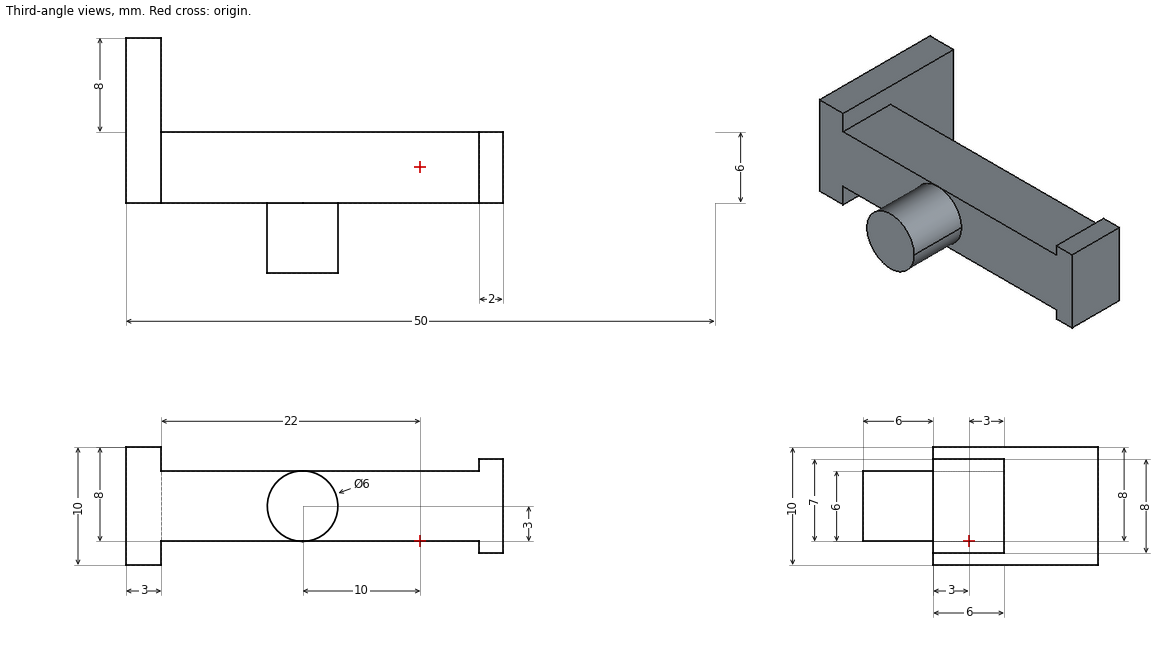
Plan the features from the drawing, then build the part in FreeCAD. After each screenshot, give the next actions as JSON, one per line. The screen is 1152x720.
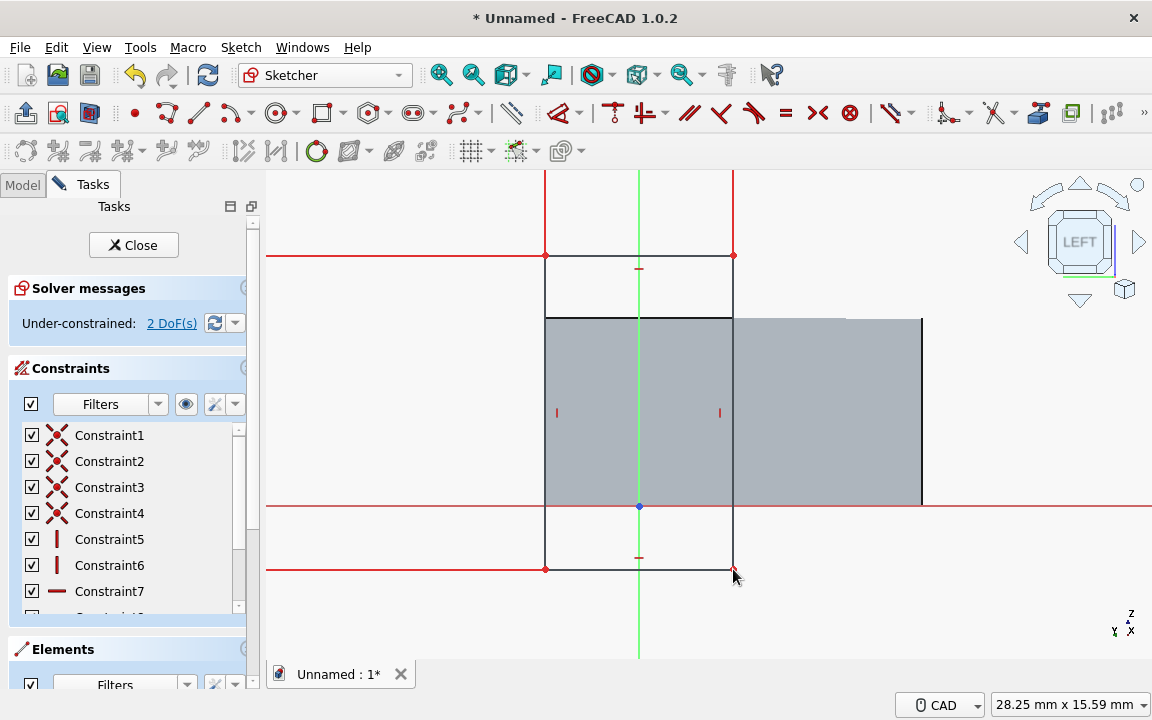
{"action": "left_click", "coordinate": [558, 114]}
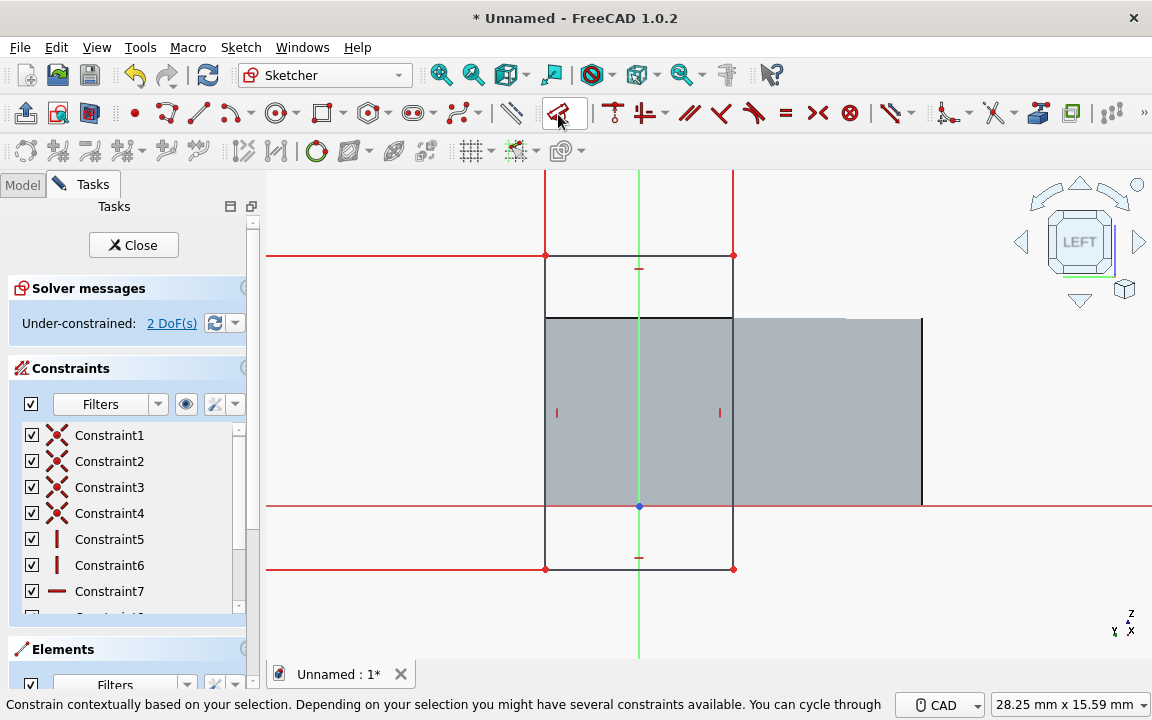
{"action": "left_click", "coordinate": [545, 256]}
{"action": "left_click", "coordinate": [592, 222]}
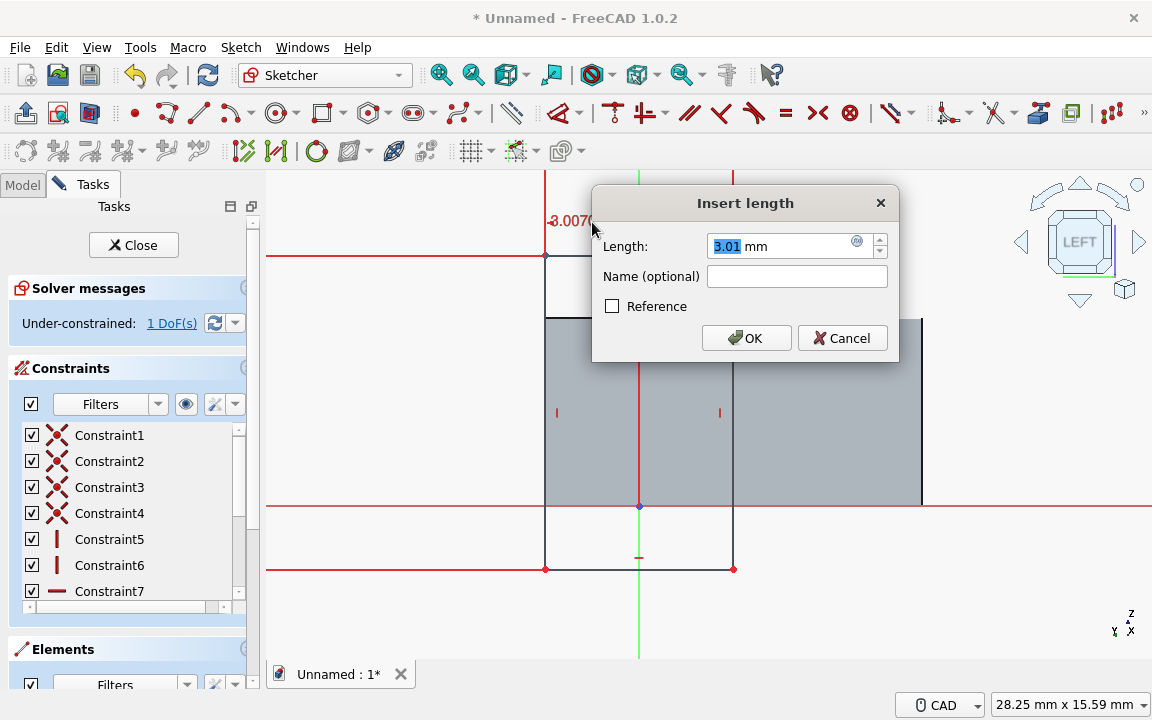
{"action": "type", "text": "3"}
{"action": "key", "text": "Return"}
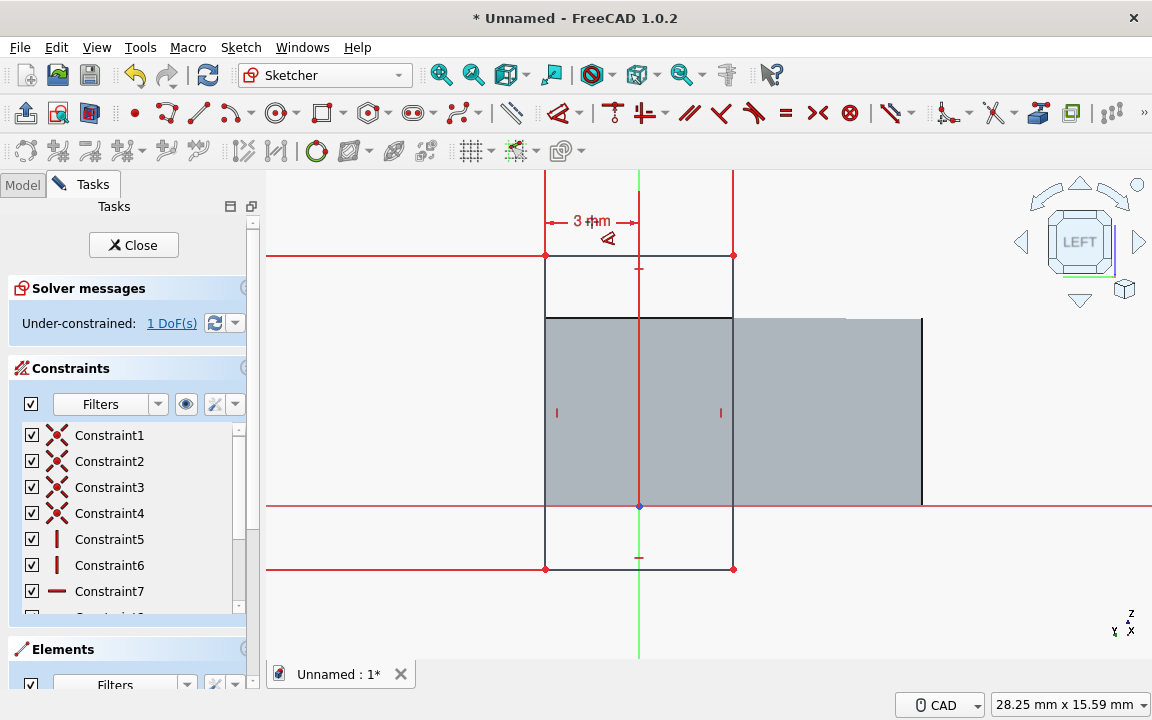
{"action": "left_click", "coordinate": [545, 256]}
{"action": "left_click", "coordinate": [511, 381]}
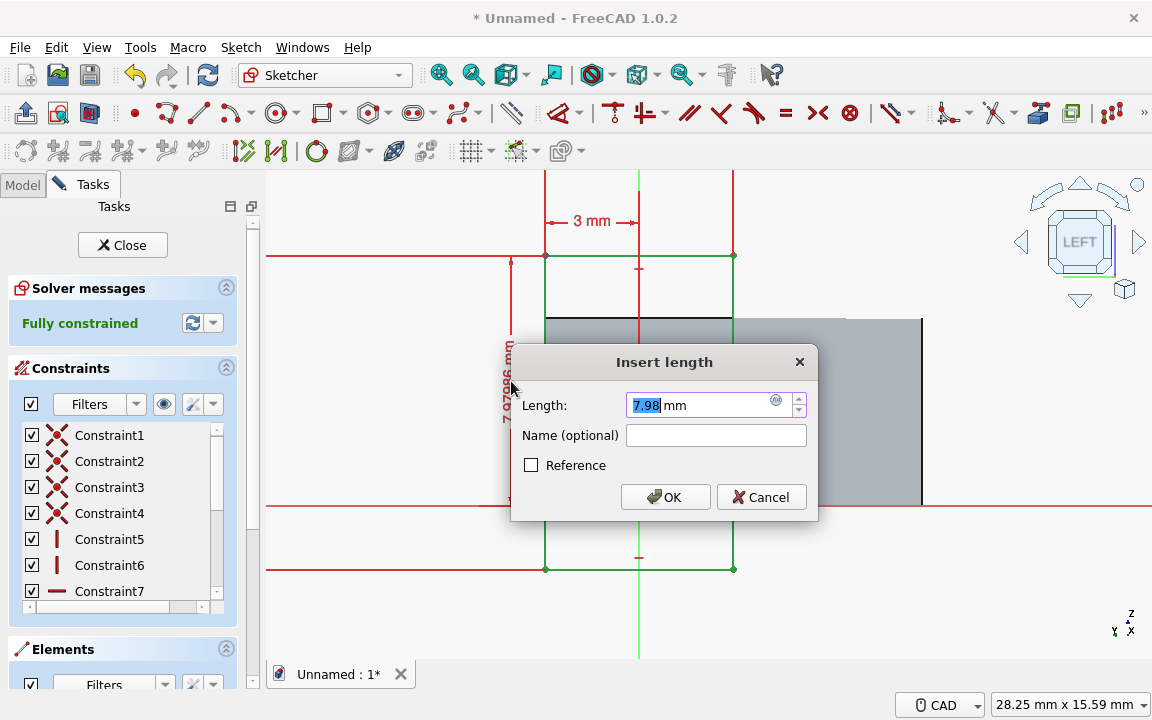
{"action": "type", "text": "8"}
{"action": "key", "text": "Return"}
{"action": "key", "text": "Escape"}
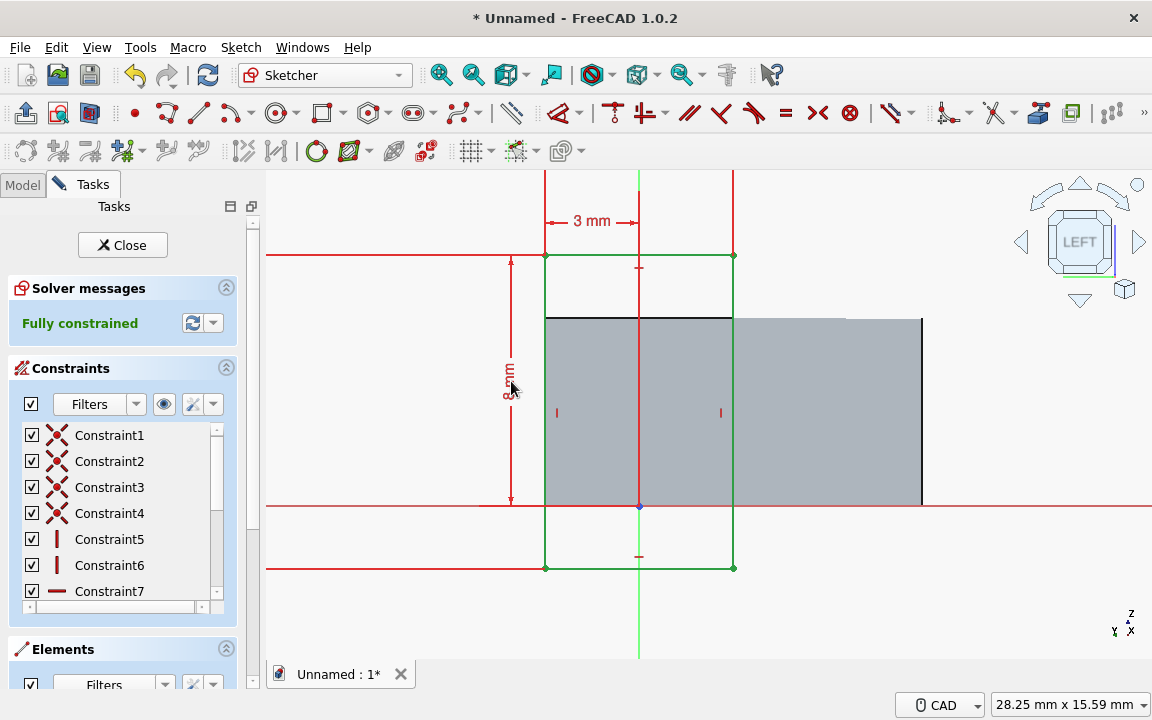
{"action": "left_click", "coordinate": [123, 245]}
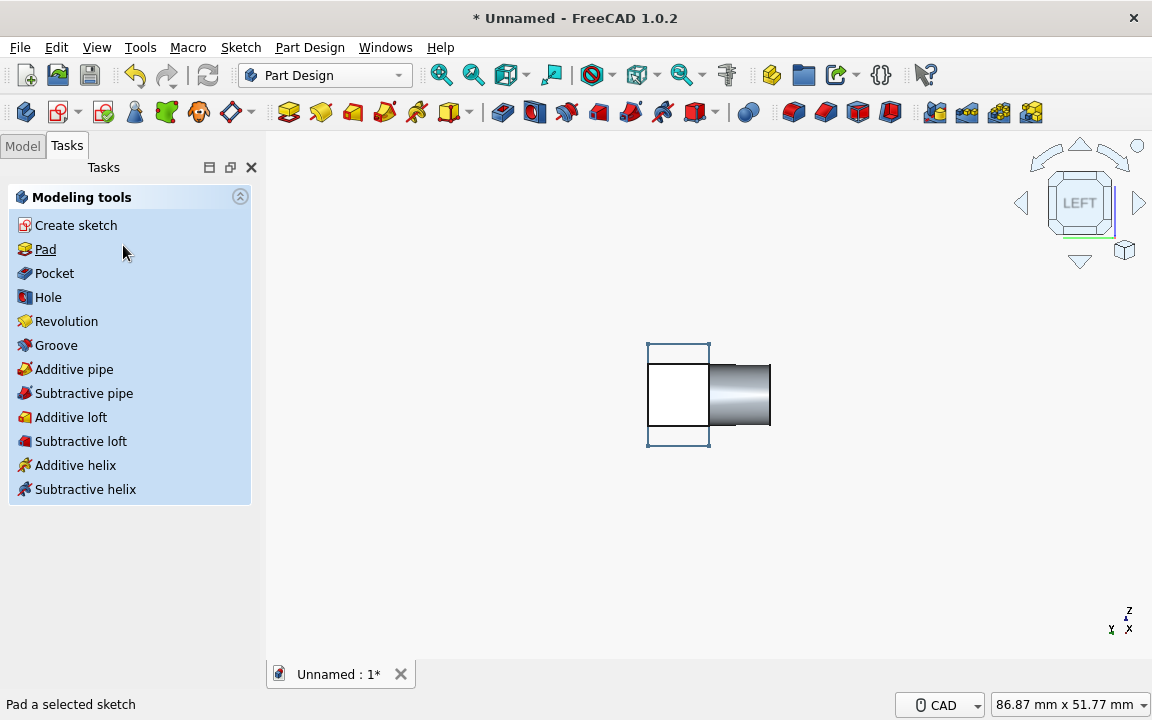
{"action": "left_click", "coordinate": [290, 112]}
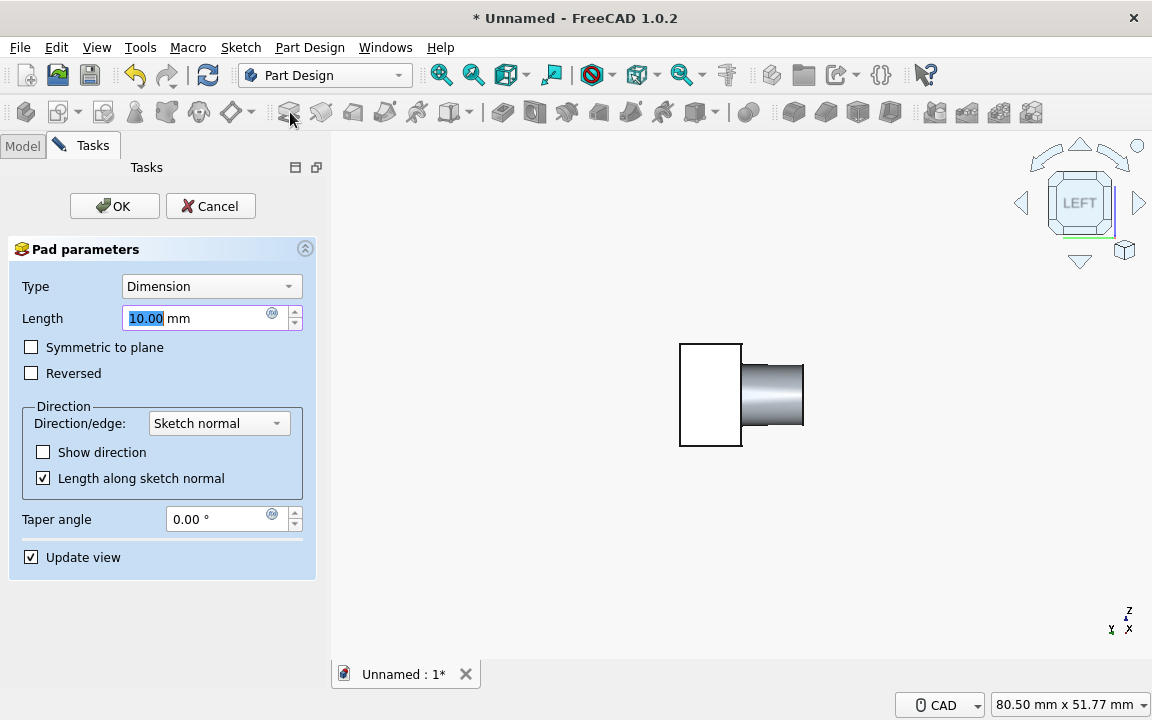
{"action": "type", "text": "3"}
{"action": "key", "text": "Tab"}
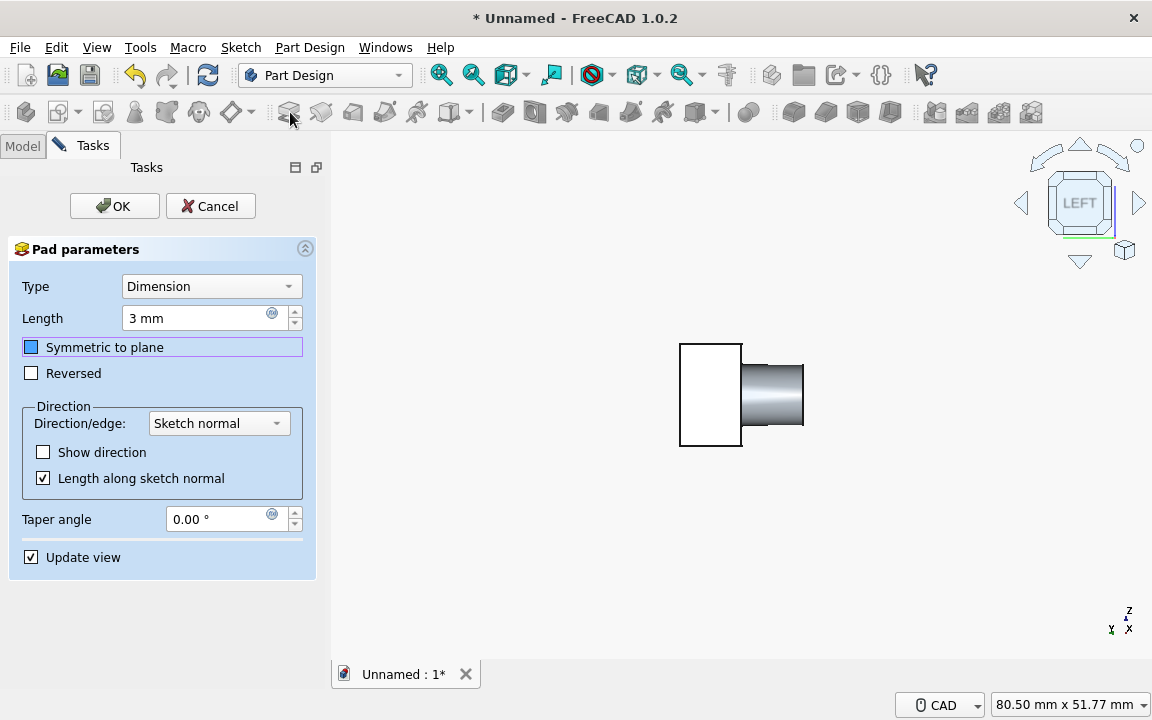
{"action": "left_click", "coordinate": [30, 373]}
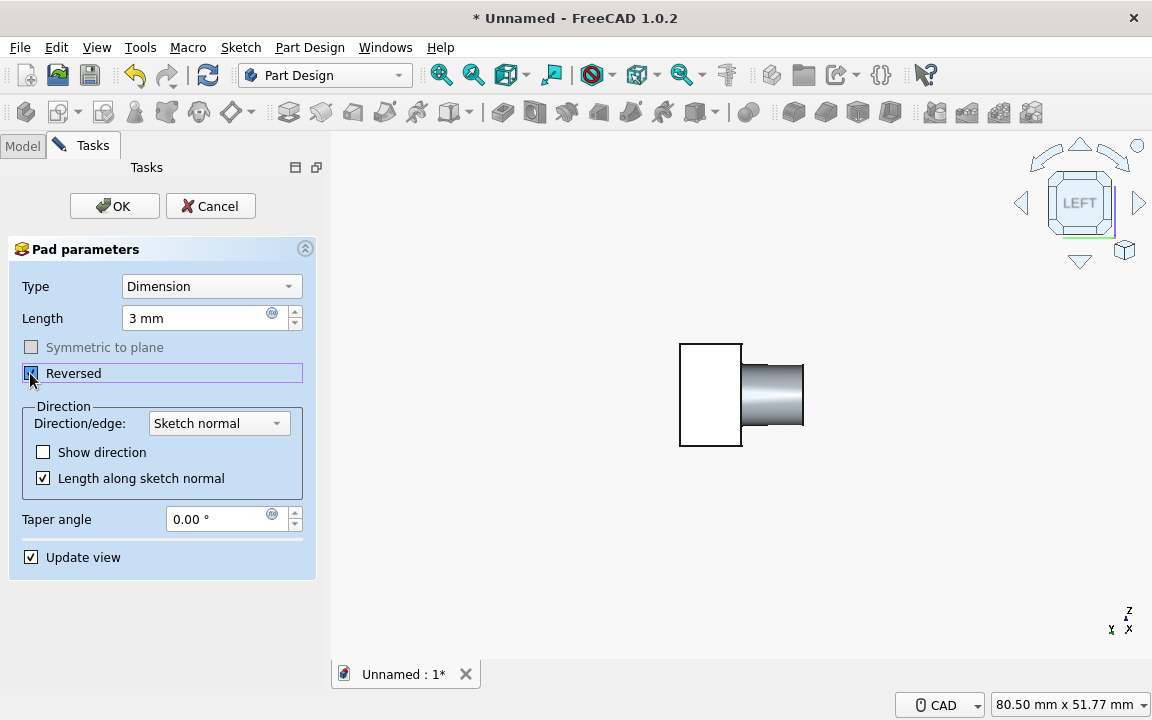
{"action": "left_click", "coordinate": [115, 206]}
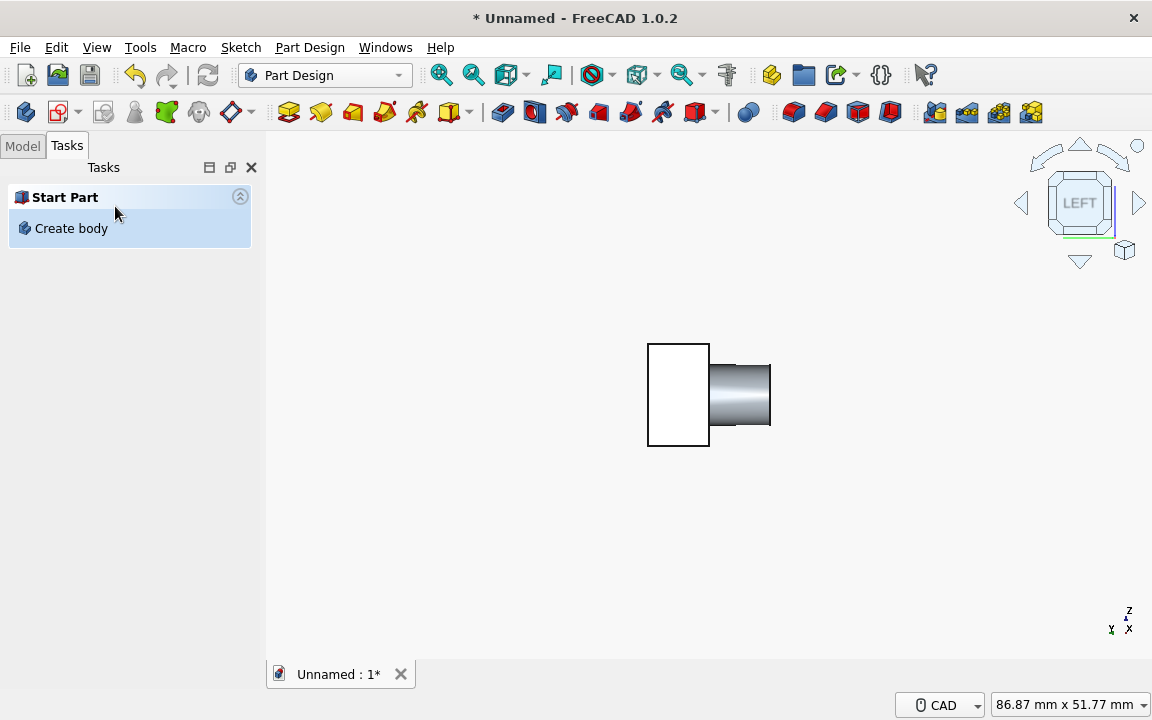
{"action": "left_click", "coordinate": [442, 76]}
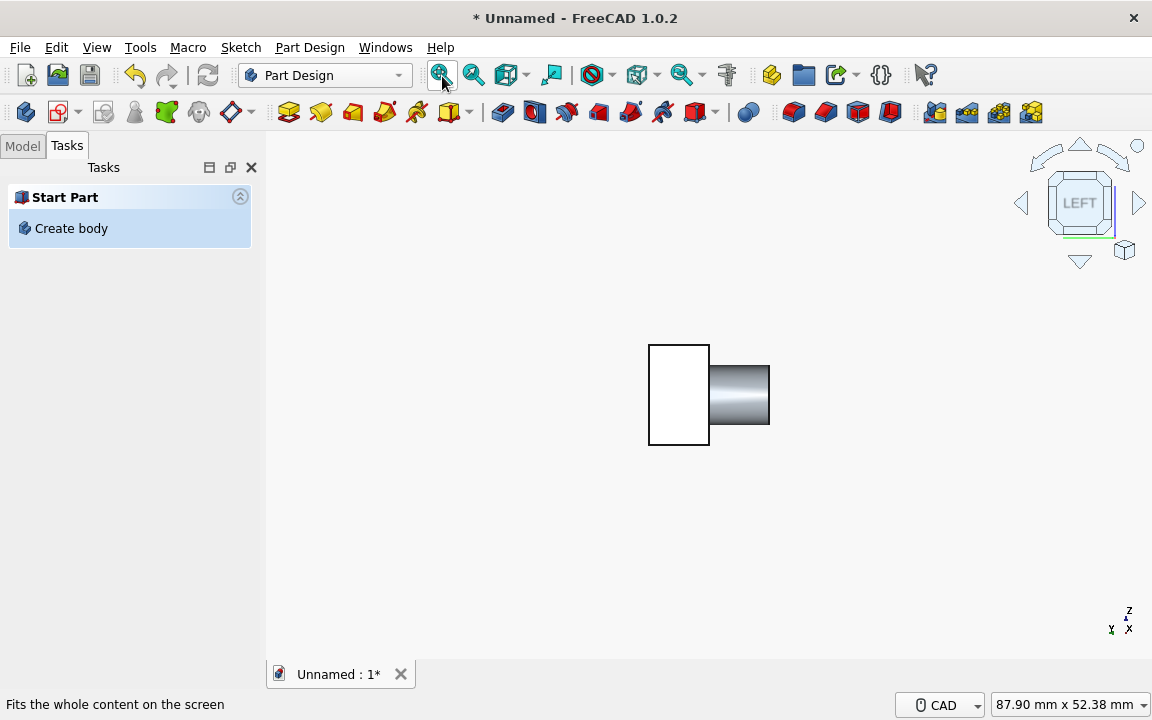
{"action": "key", "text": "0"}